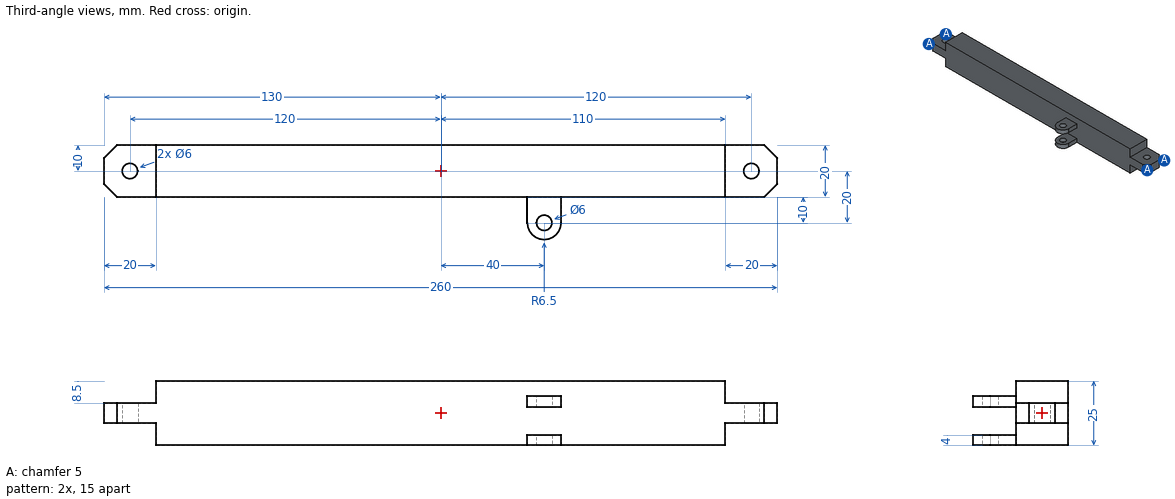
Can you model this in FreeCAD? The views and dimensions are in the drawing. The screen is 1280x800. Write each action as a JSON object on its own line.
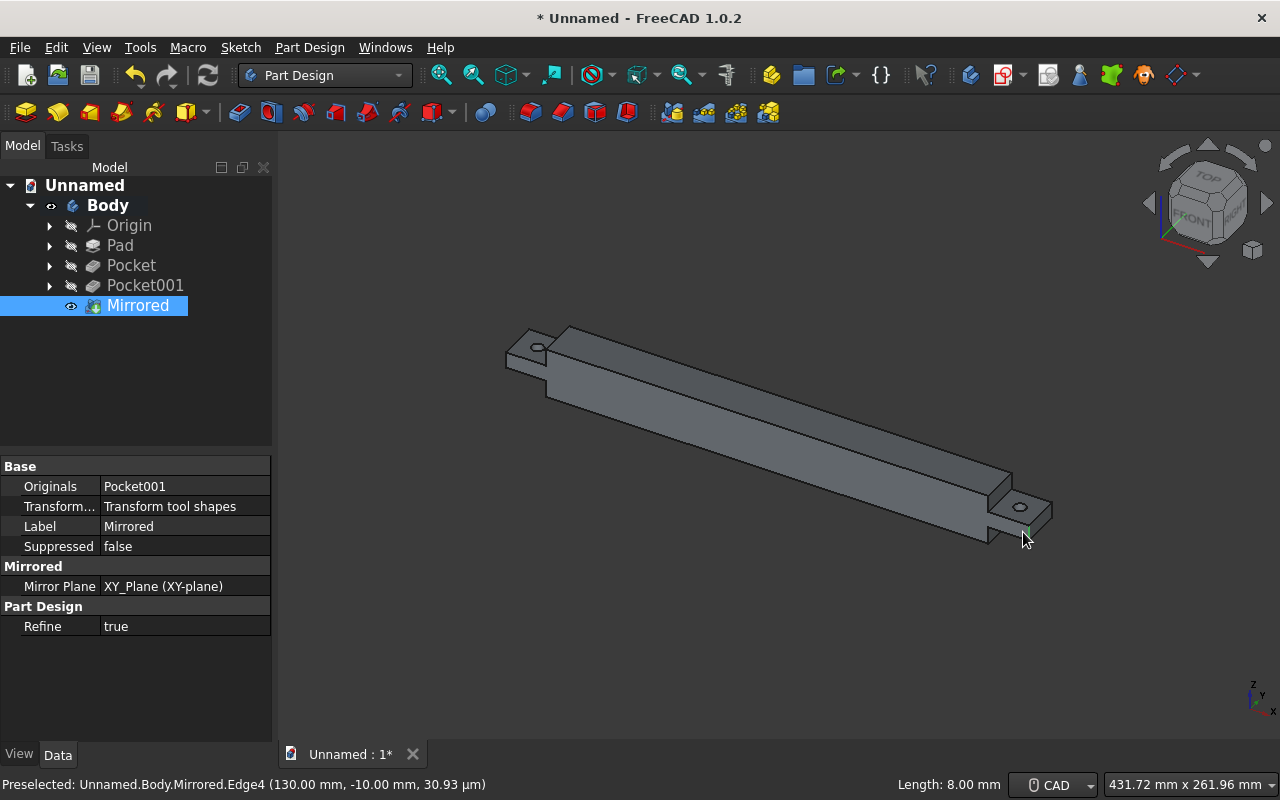
{"action": "scroll", "coordinate": [506, 359], "scroll_direction": "up", "scroll_amount": 4}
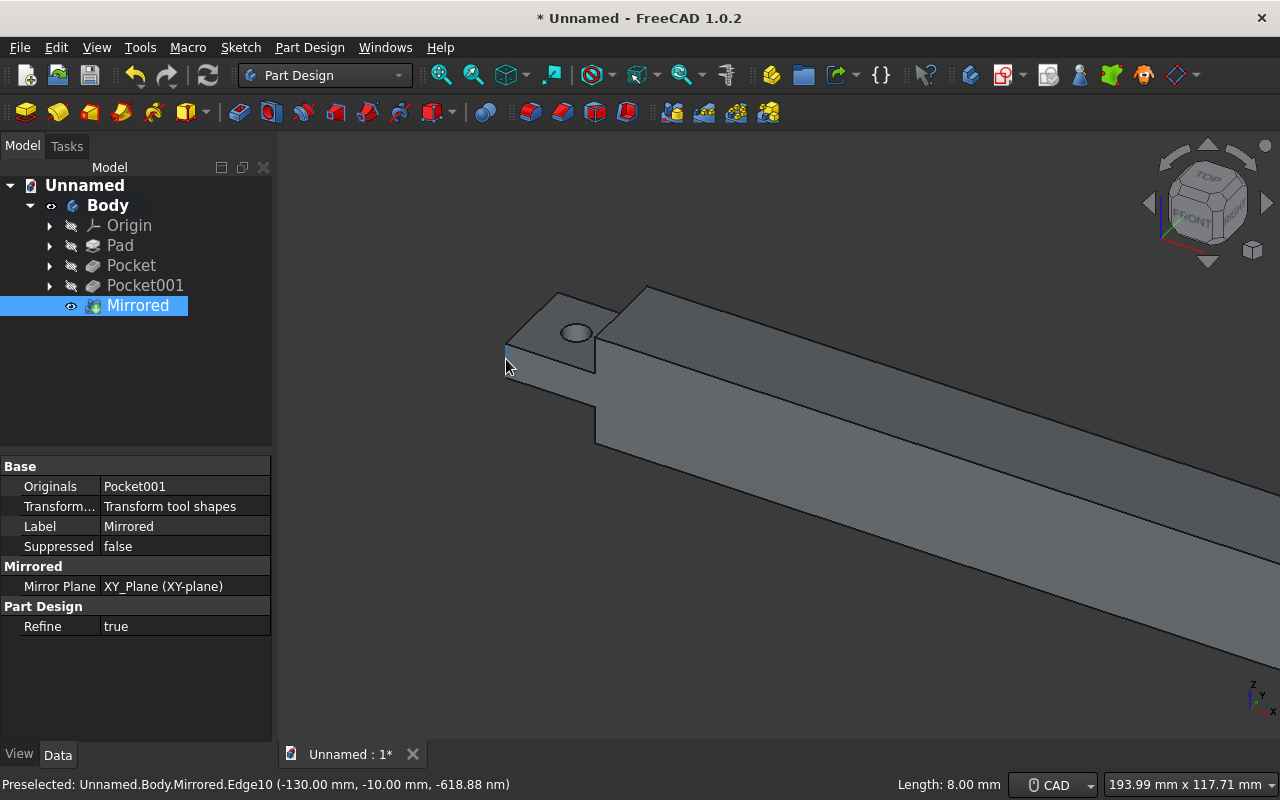
{"action": "left_click", "coordinate": [442, 76]}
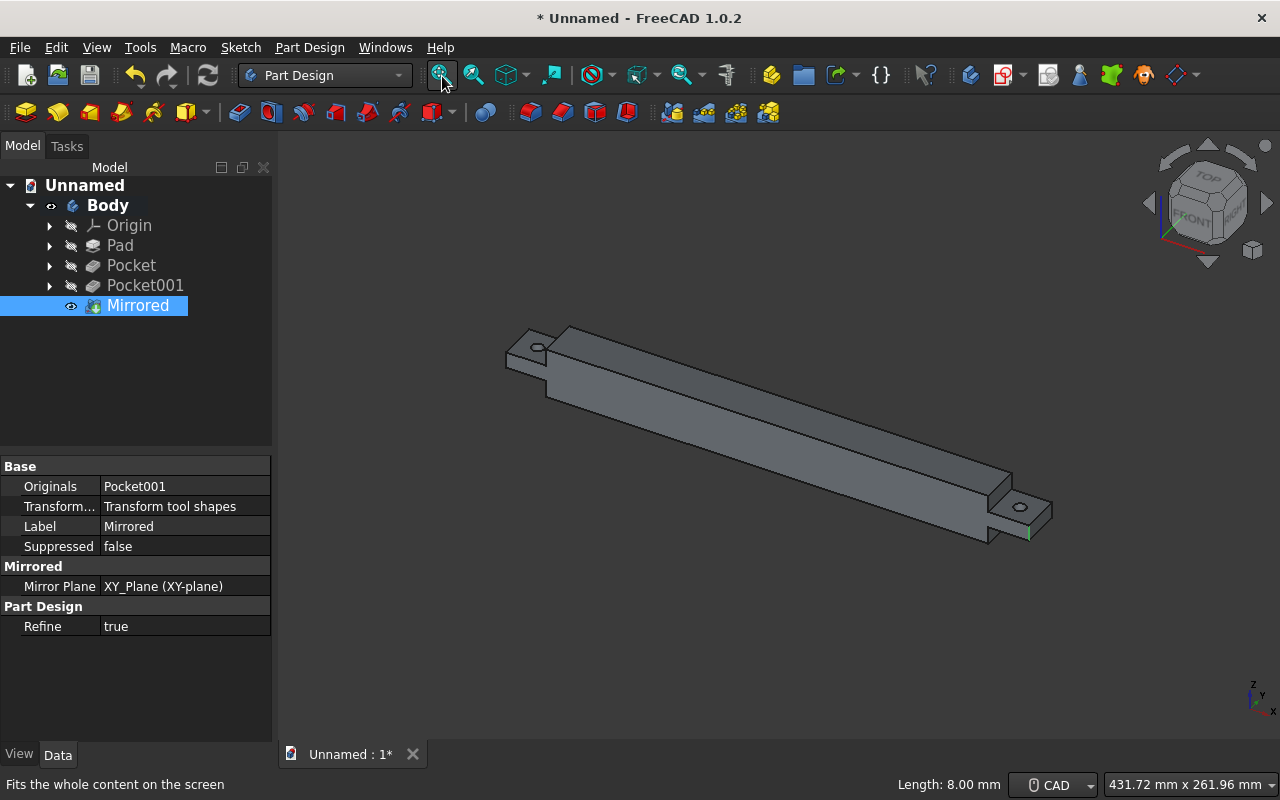
{"action": "key", "text": "0"}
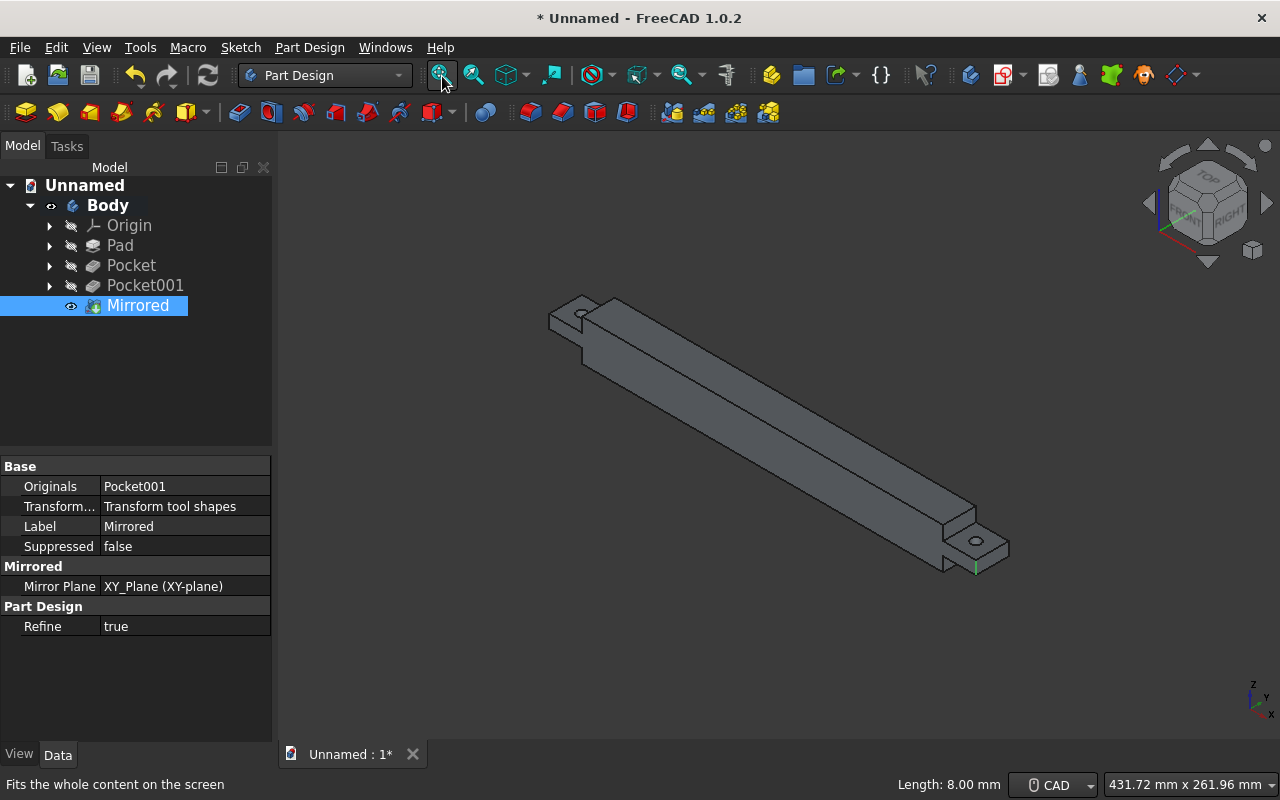
{"action": "scroll", "coordinate": [549, 320], "scroll_direction": "up", "scroll_amount": 4}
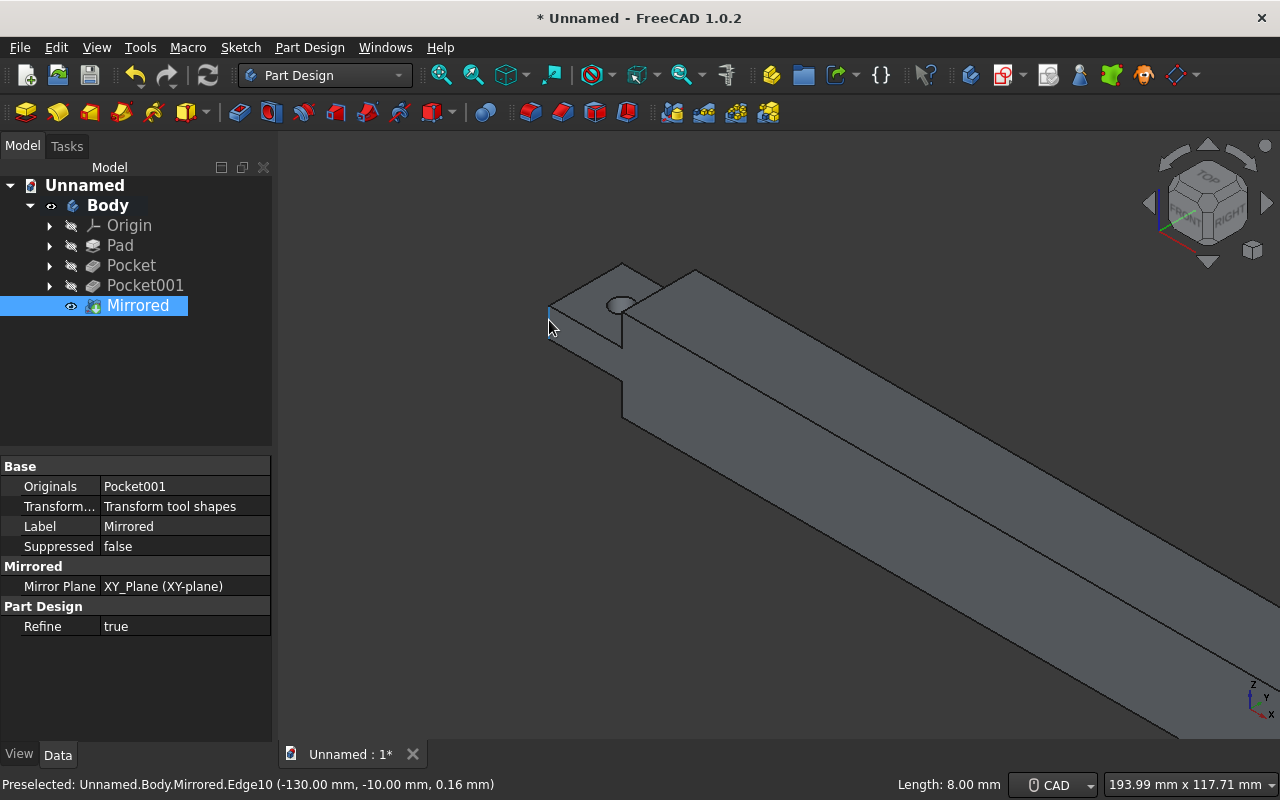
{"action": "key", "text": "v f"}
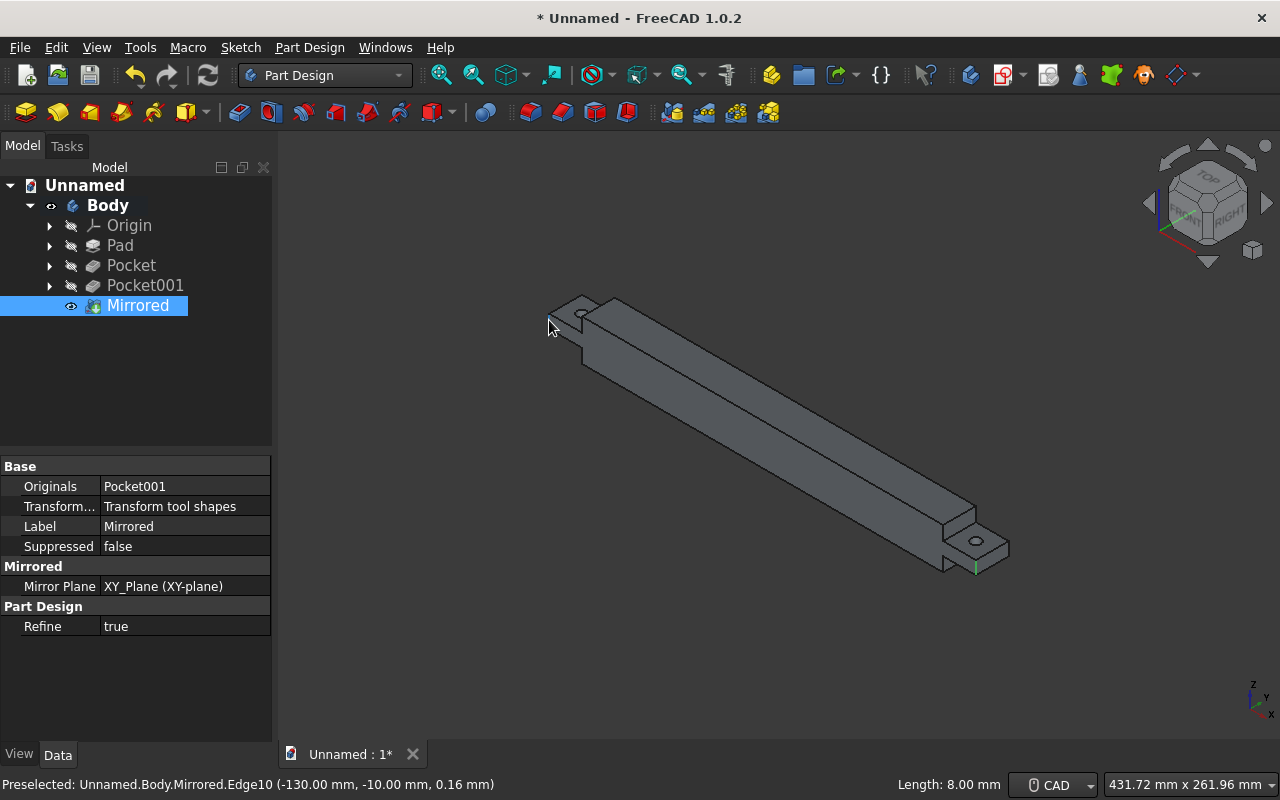
{"action": "key", "text": "2"}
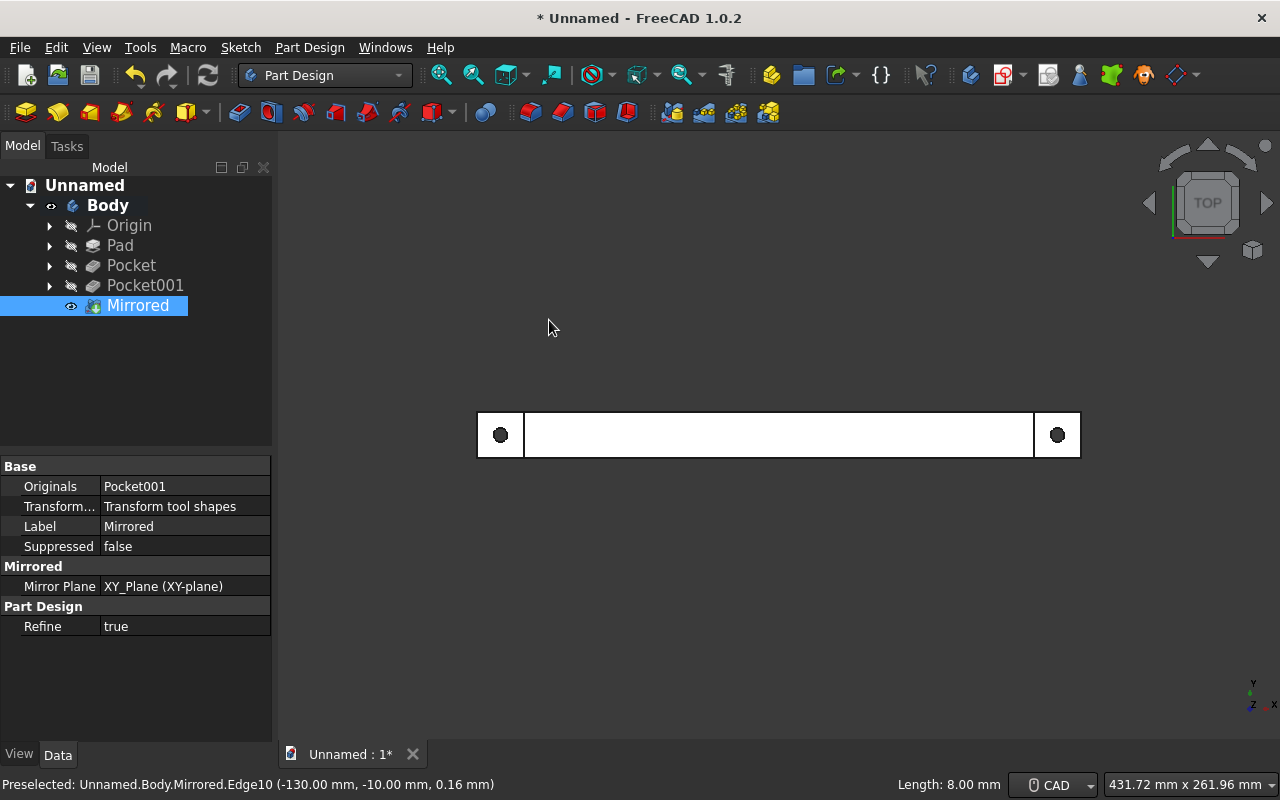
{"action": "scroll", "coordinate": [477, 457], "scroll_direction": "up", "scroll_amount": 4}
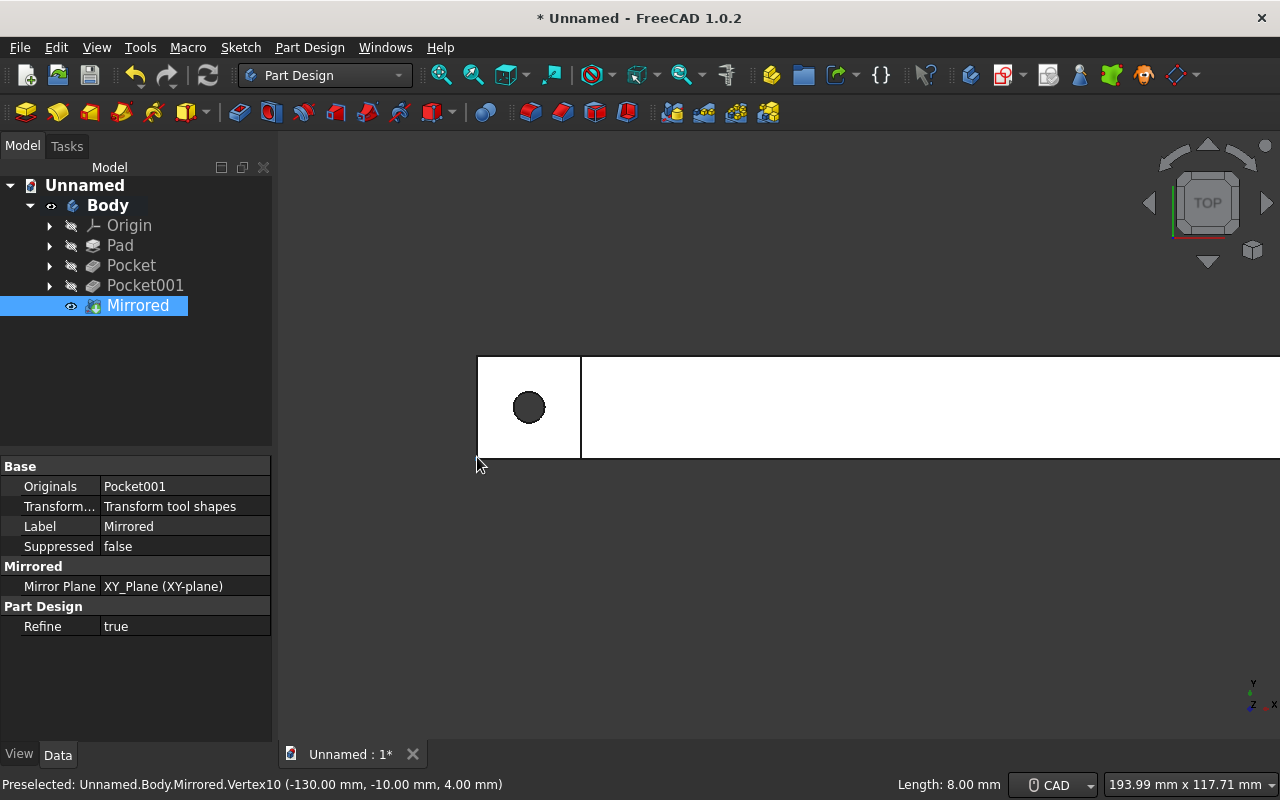
{"action": "key", "text": "v f"}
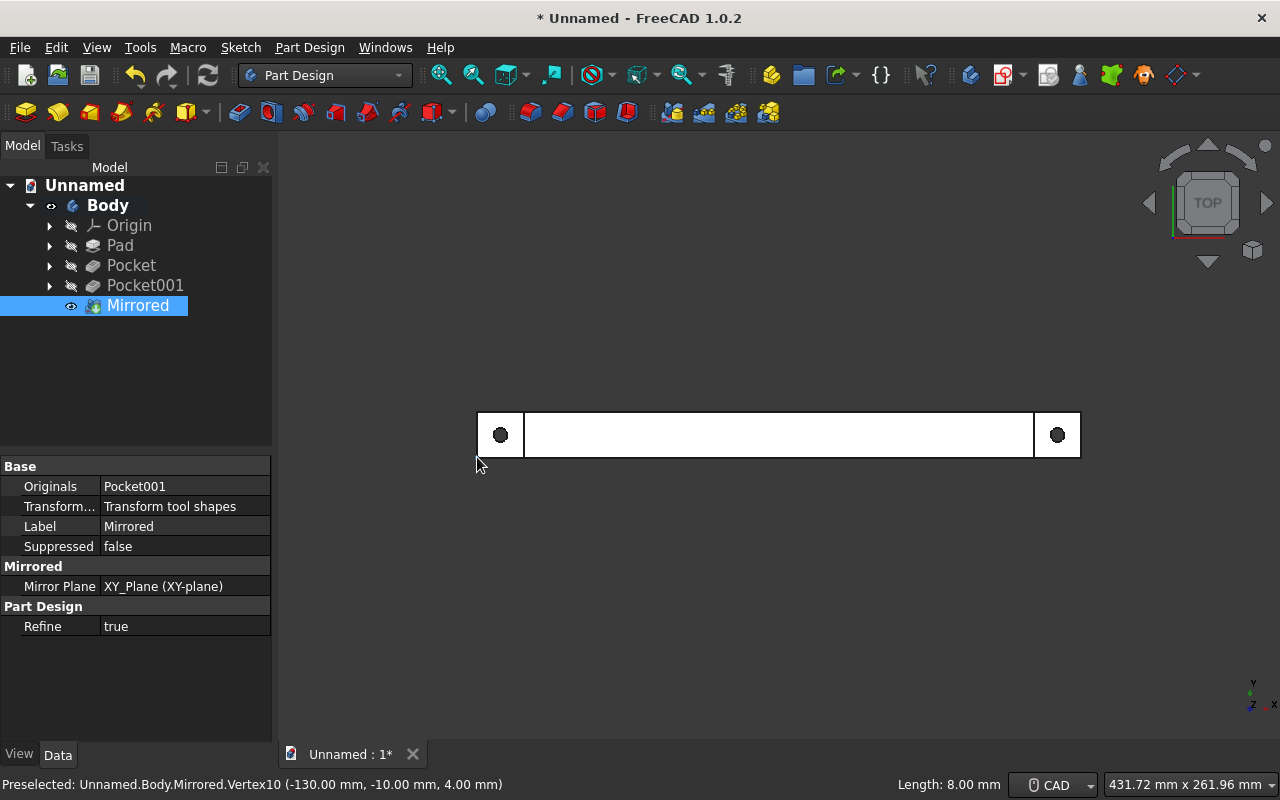
{"action": "key", "text": "1"}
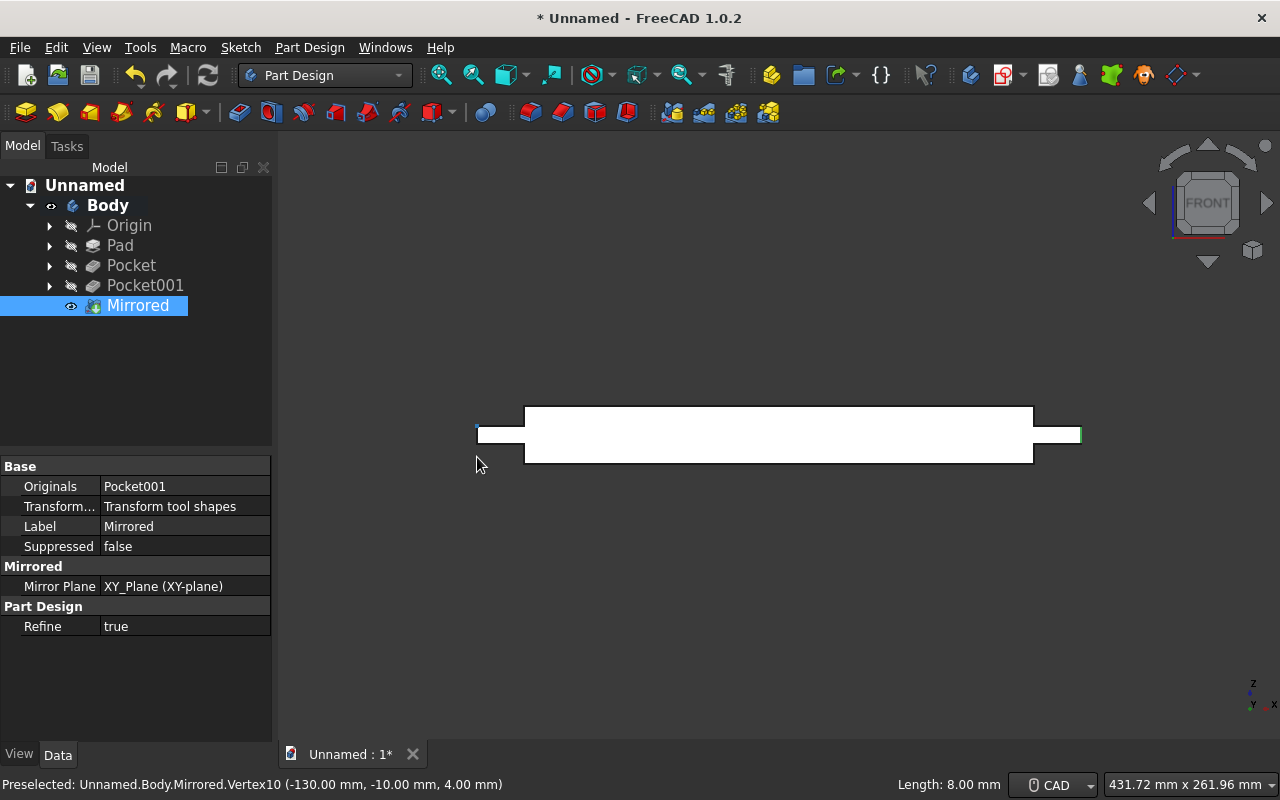
{"action": "left_click", "coordinate": [477, 434], "text": "ctrl"}